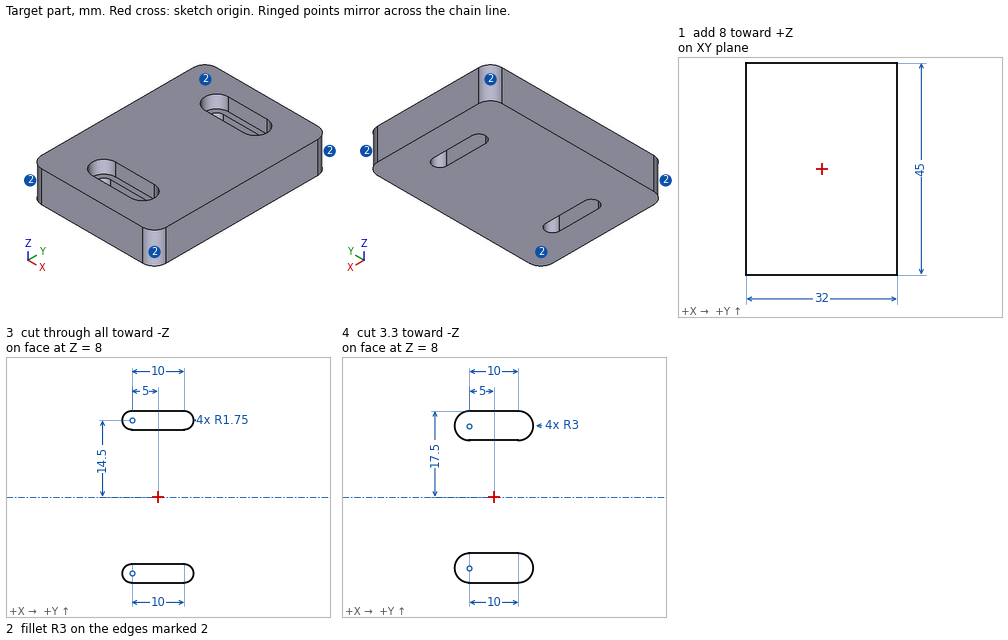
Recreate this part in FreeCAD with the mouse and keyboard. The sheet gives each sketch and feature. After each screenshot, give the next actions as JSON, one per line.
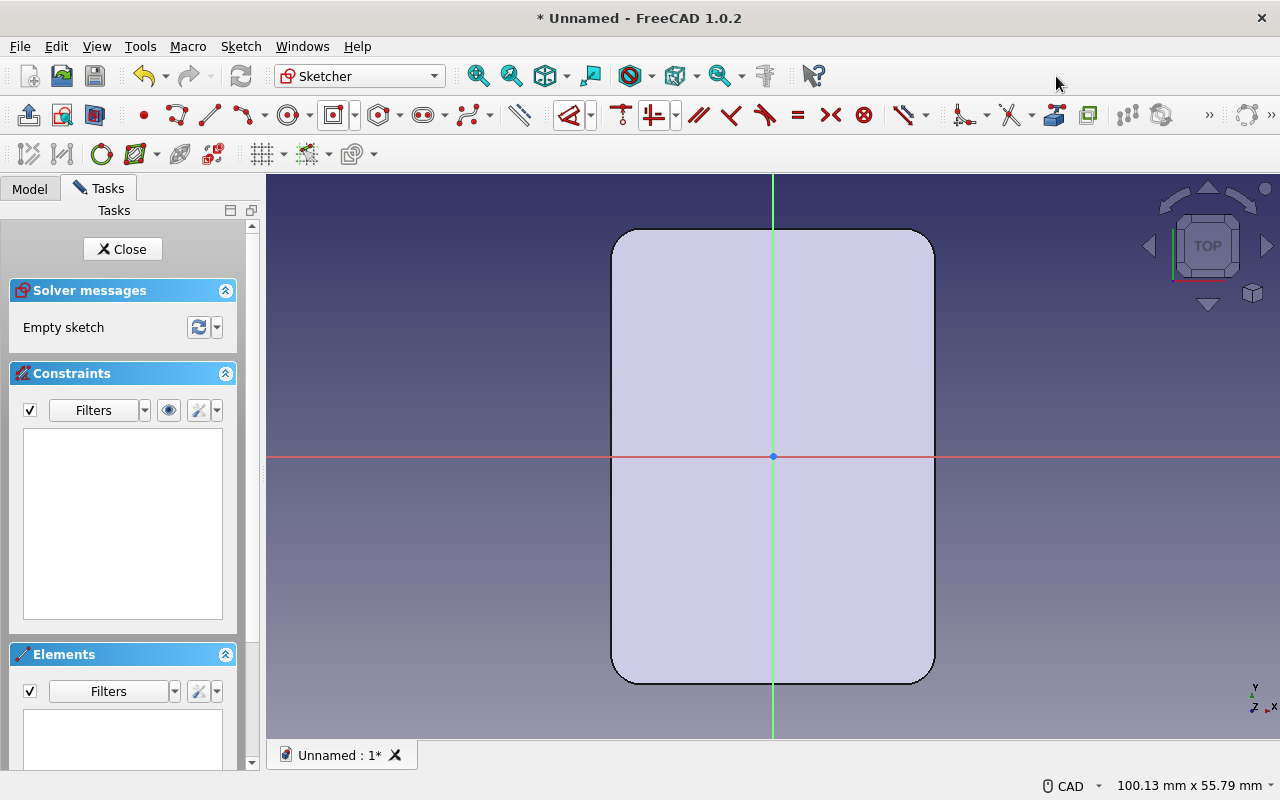
{"action": "left_click", "coordinate": [422, 116]}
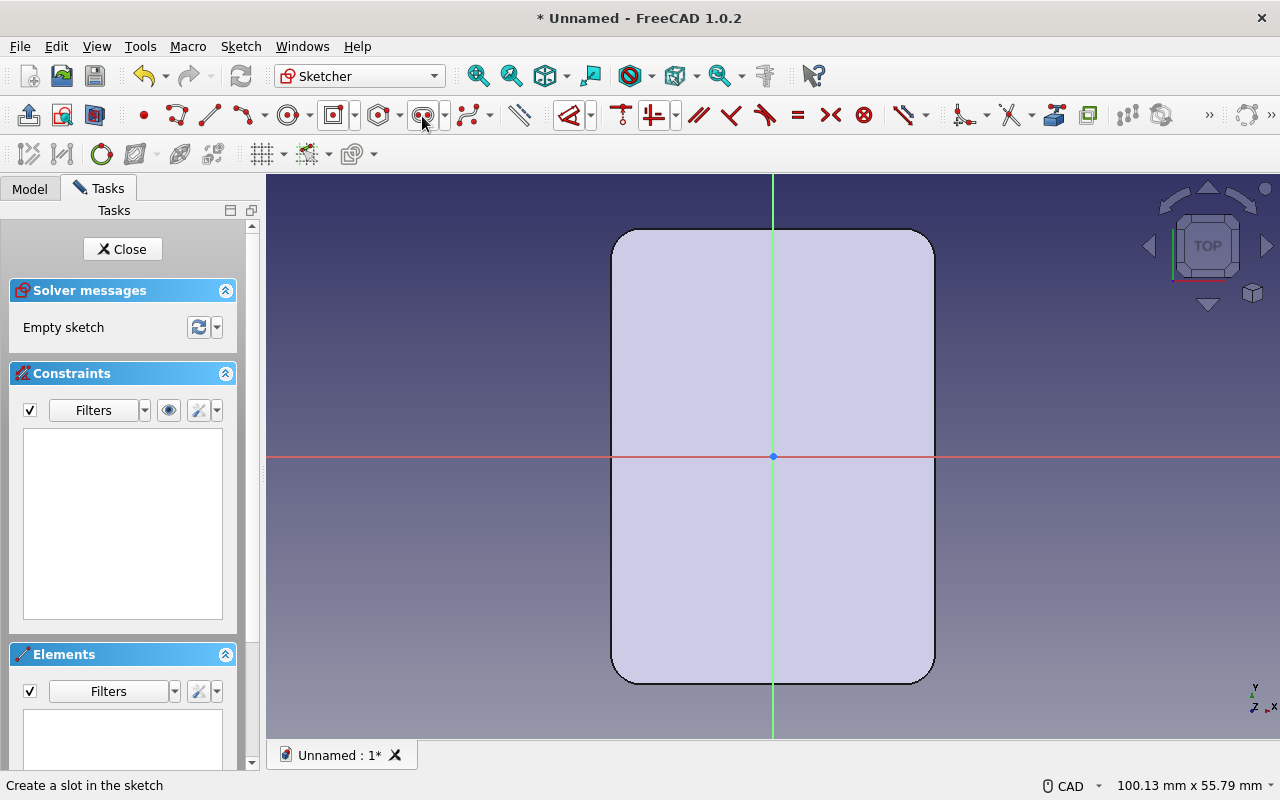
{"action": "scroll", "coordinate": [722, 310], "scroll_direction": "up", "scroll_amount": 2}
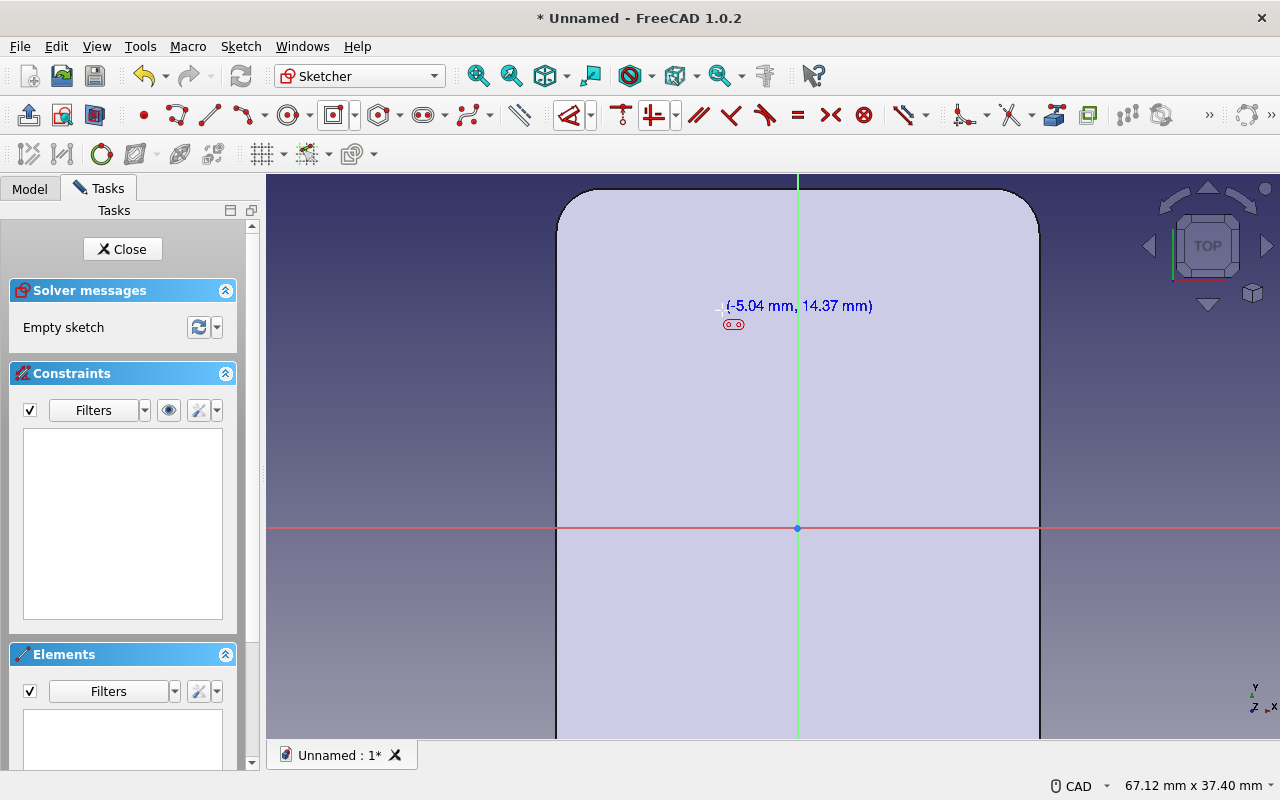
{"action": "left_click", "coordinate": [722, 309]}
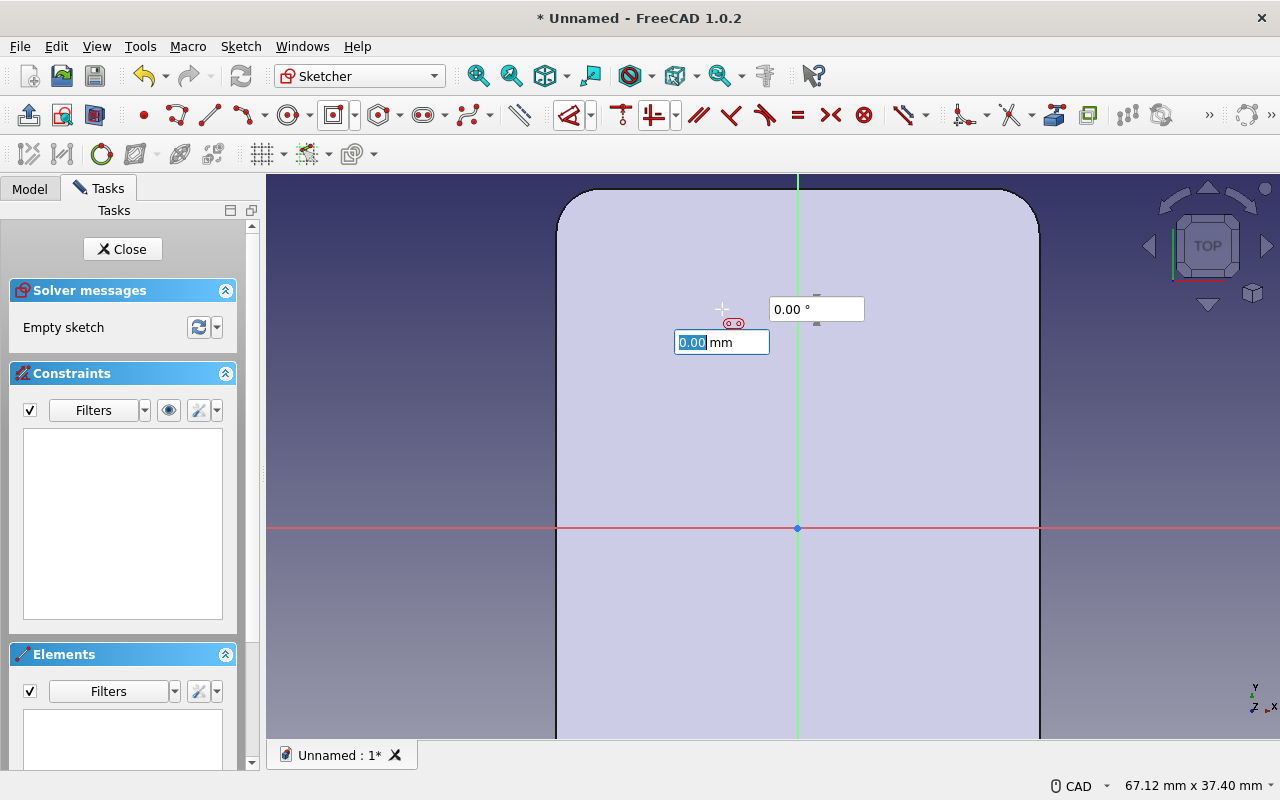
{"action": "left_click", "coordinate": [873, 309]}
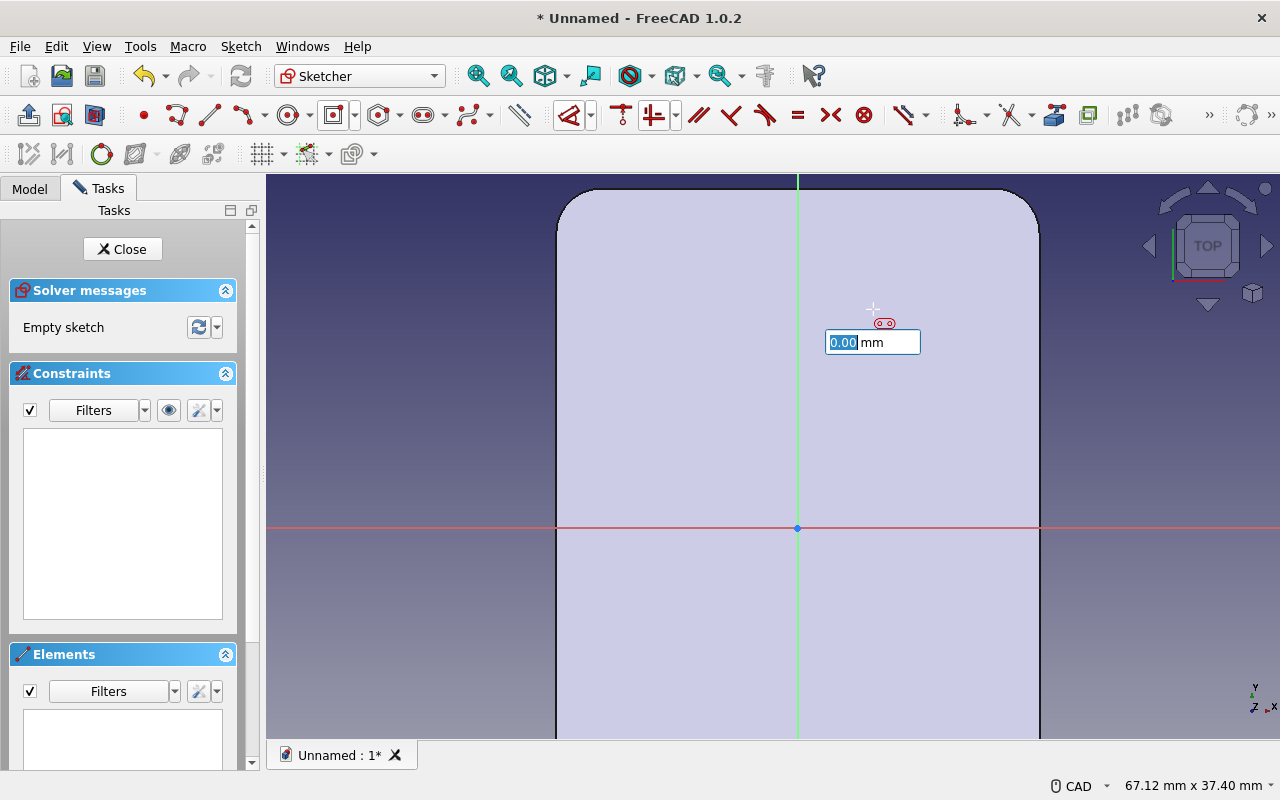
{"action": "left_click", "coordinate": [821, 283]}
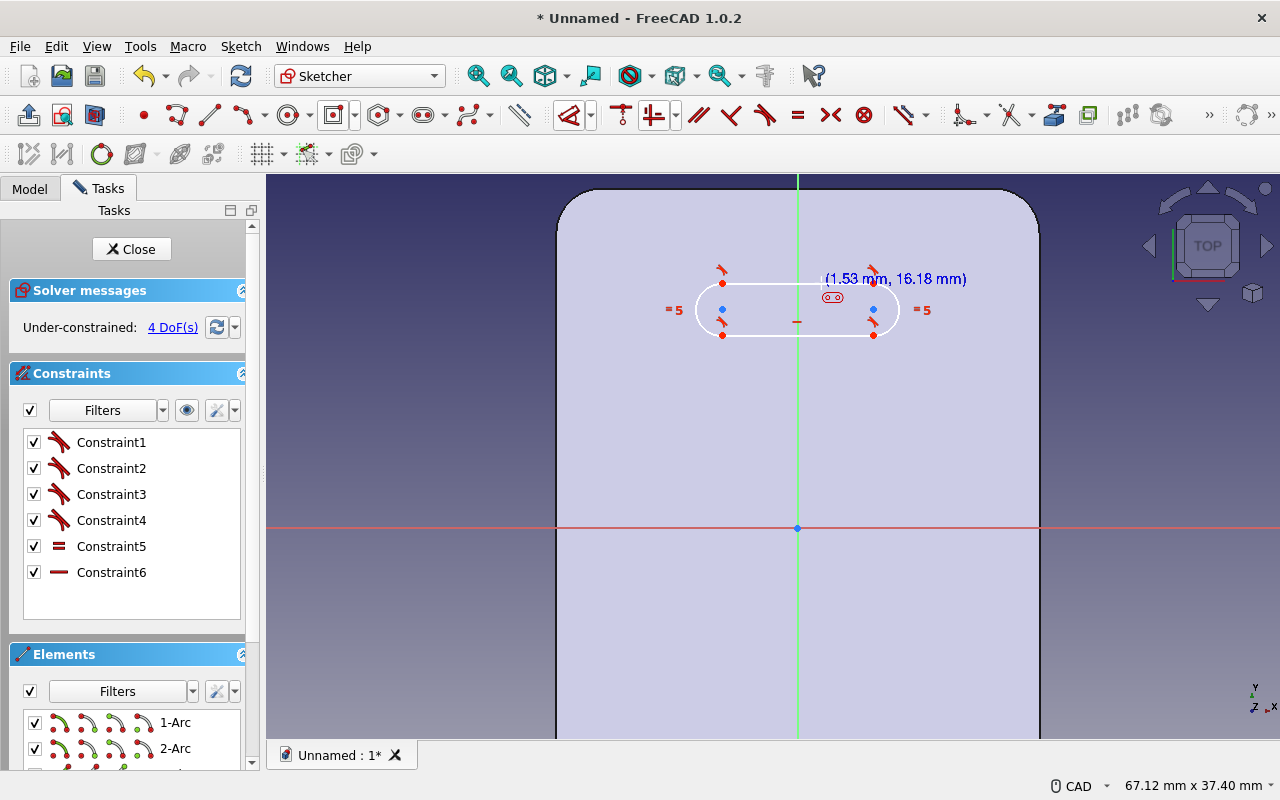
{"action": "scroll", "coordinate": [515, 310], "scroll_direction": "down", "scroll_amount": 2}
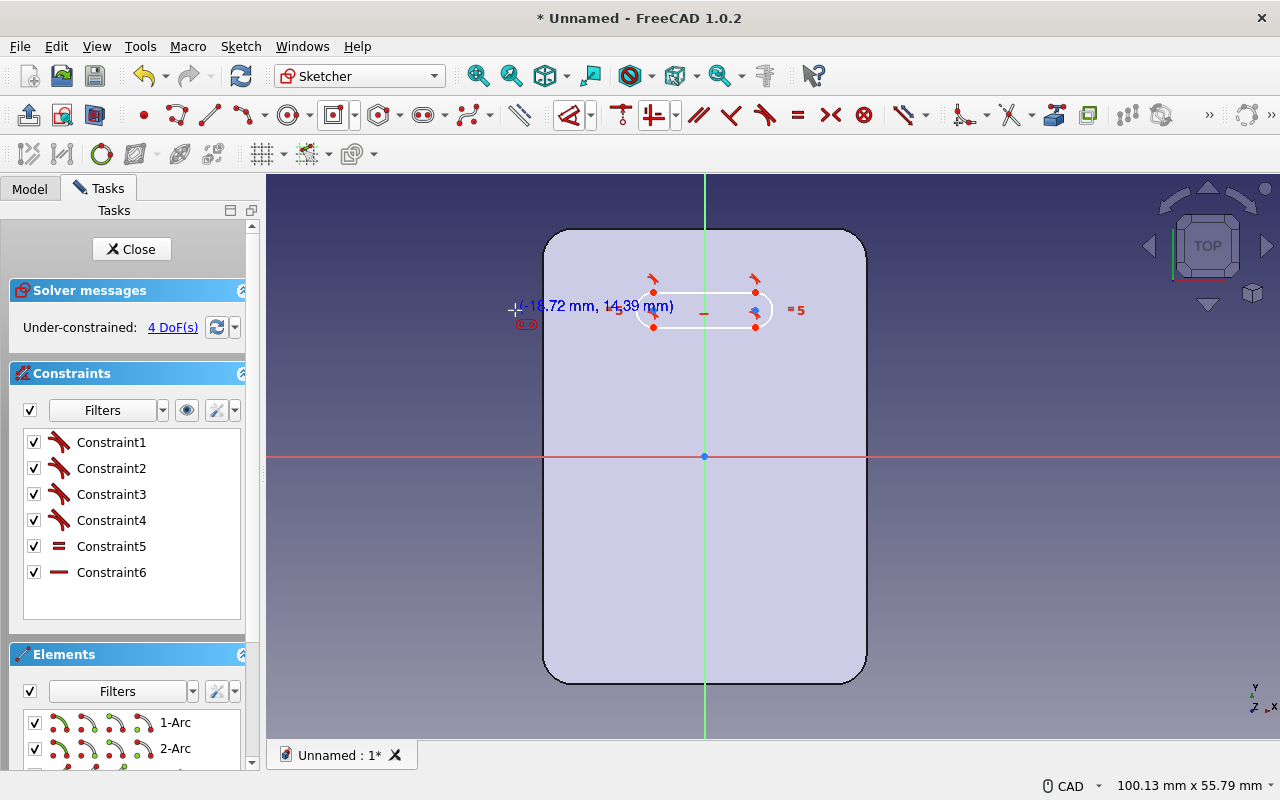
{"action": "scroll", "coordinate": [654, 603], "scroll_direction": "up", "scroll_amount": 2}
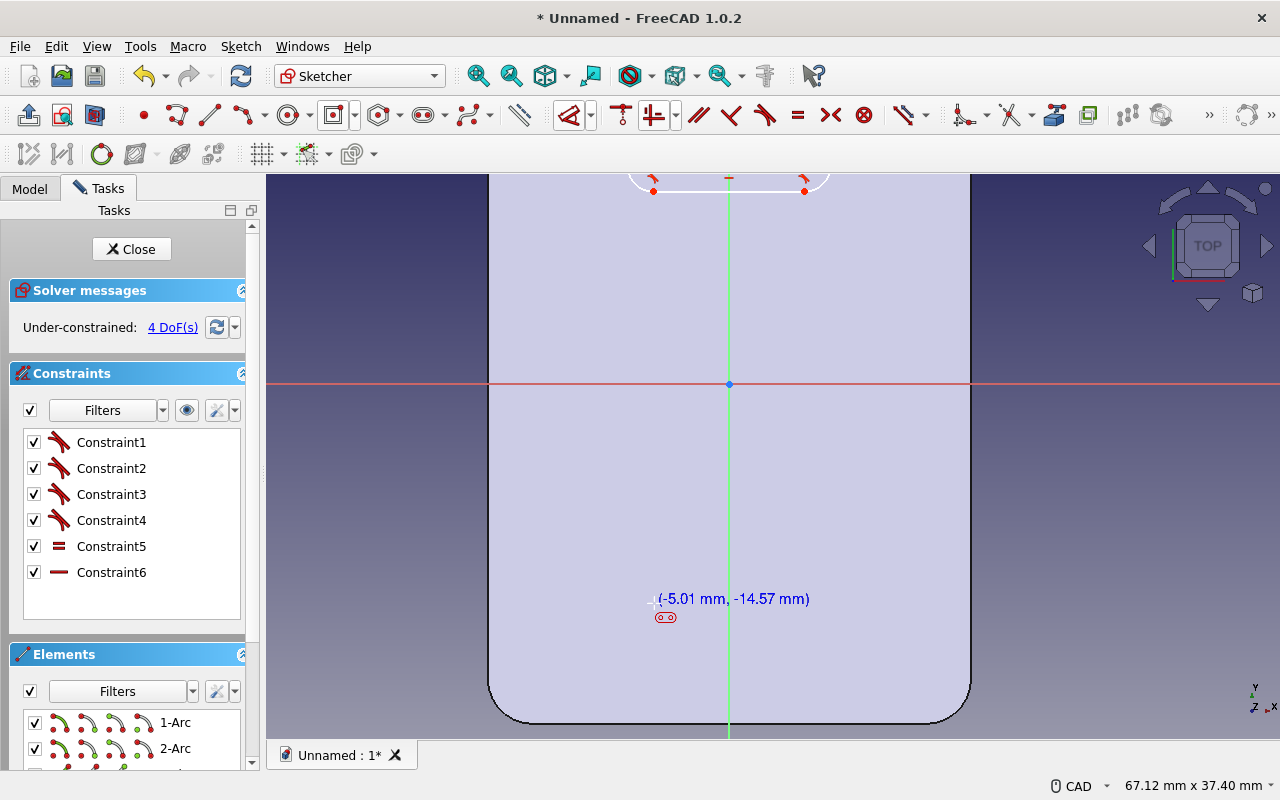
{"action": "left_click", "coordinate": [654, 603]}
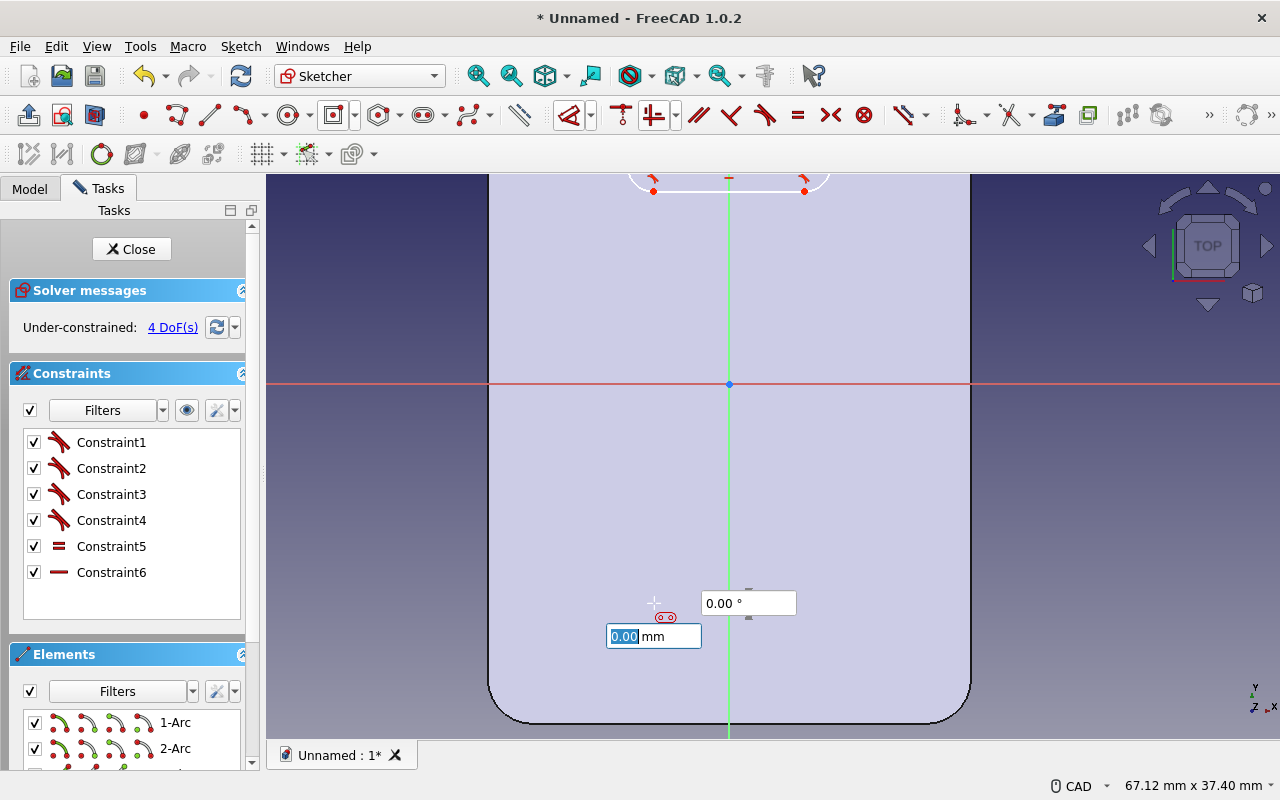
{"action": "left_click", "coordinate": [805, 603]}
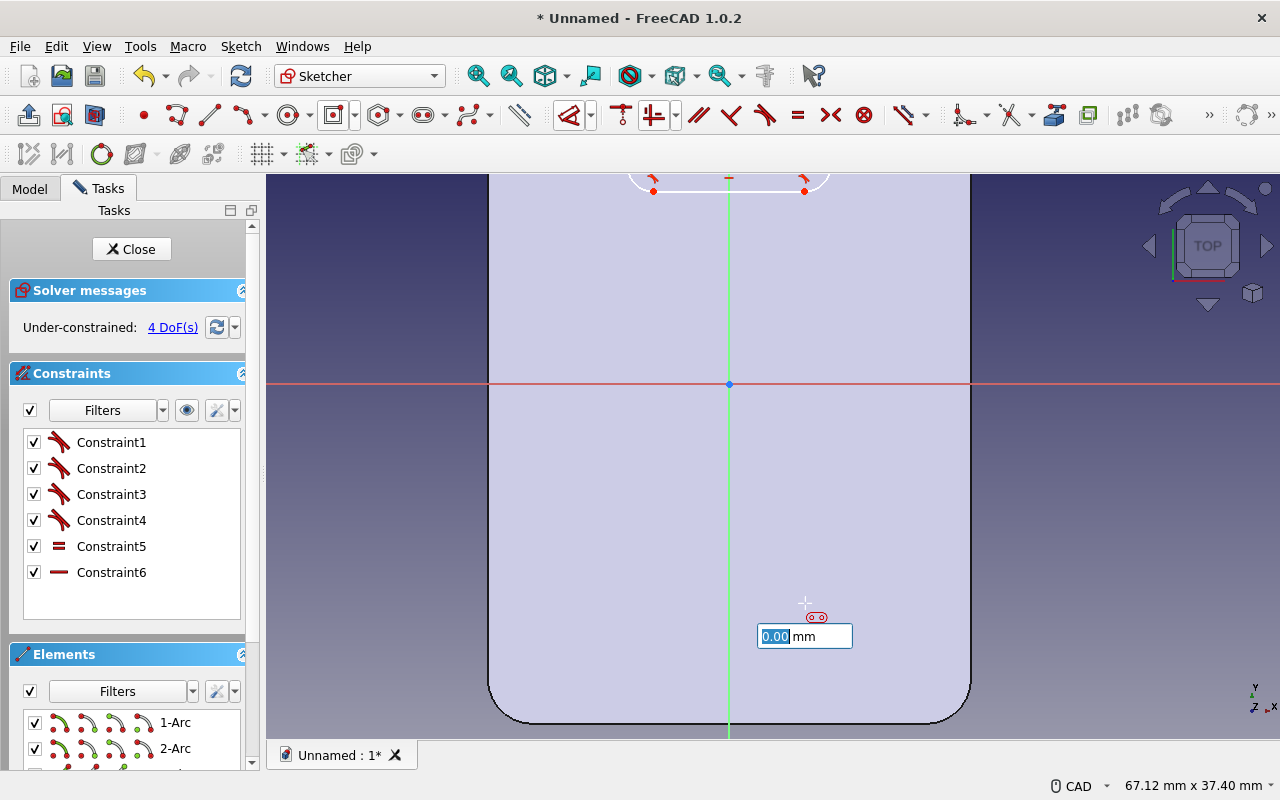
{"action": "left_click", "coordinate": [752, 577]}
{"action": "key", "text": "Escape"}